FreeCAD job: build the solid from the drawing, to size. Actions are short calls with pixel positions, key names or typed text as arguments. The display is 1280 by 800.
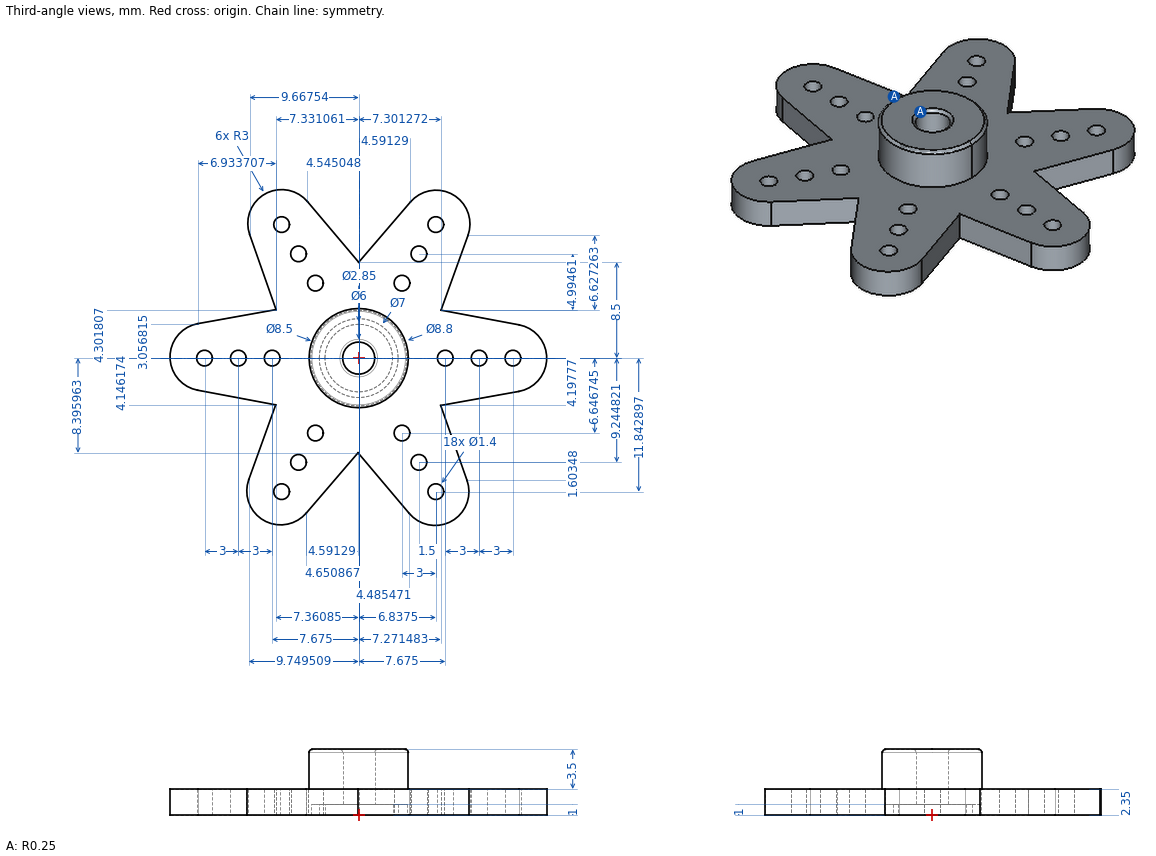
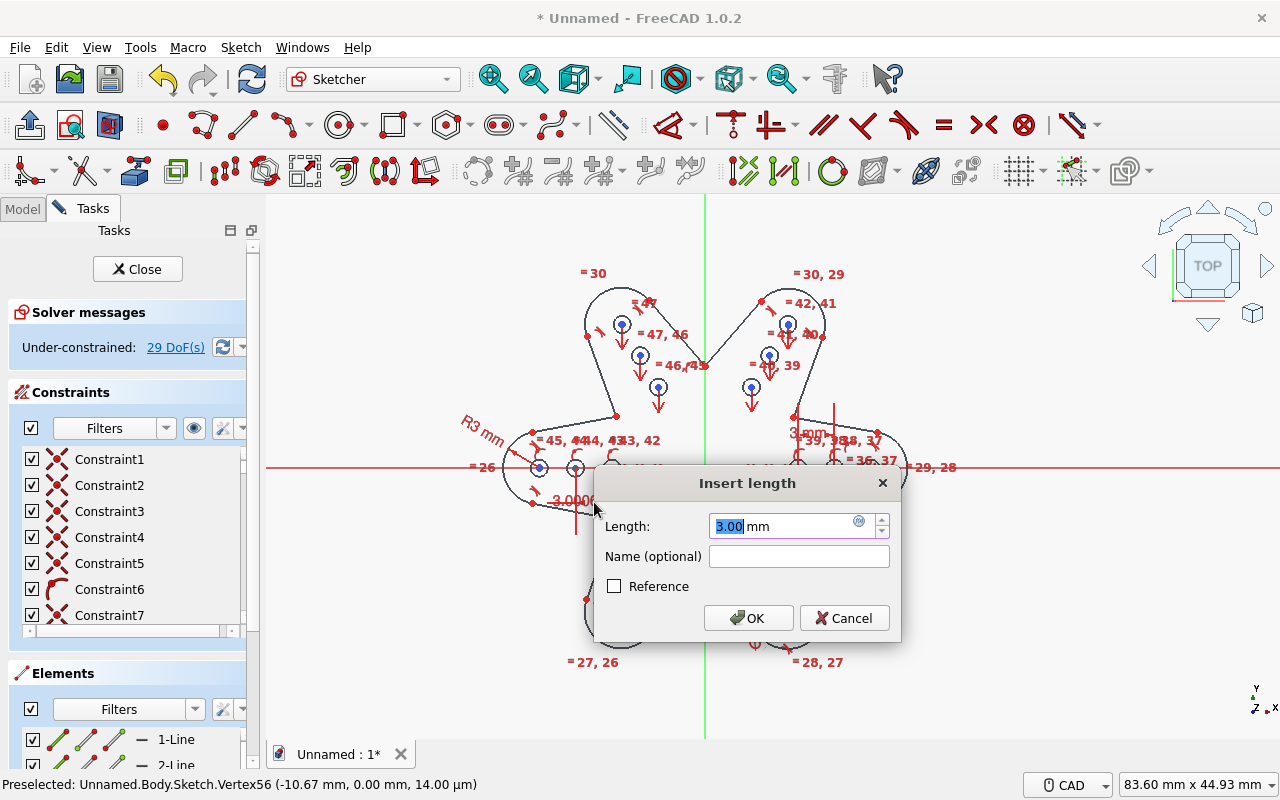
text(3)
key(Return)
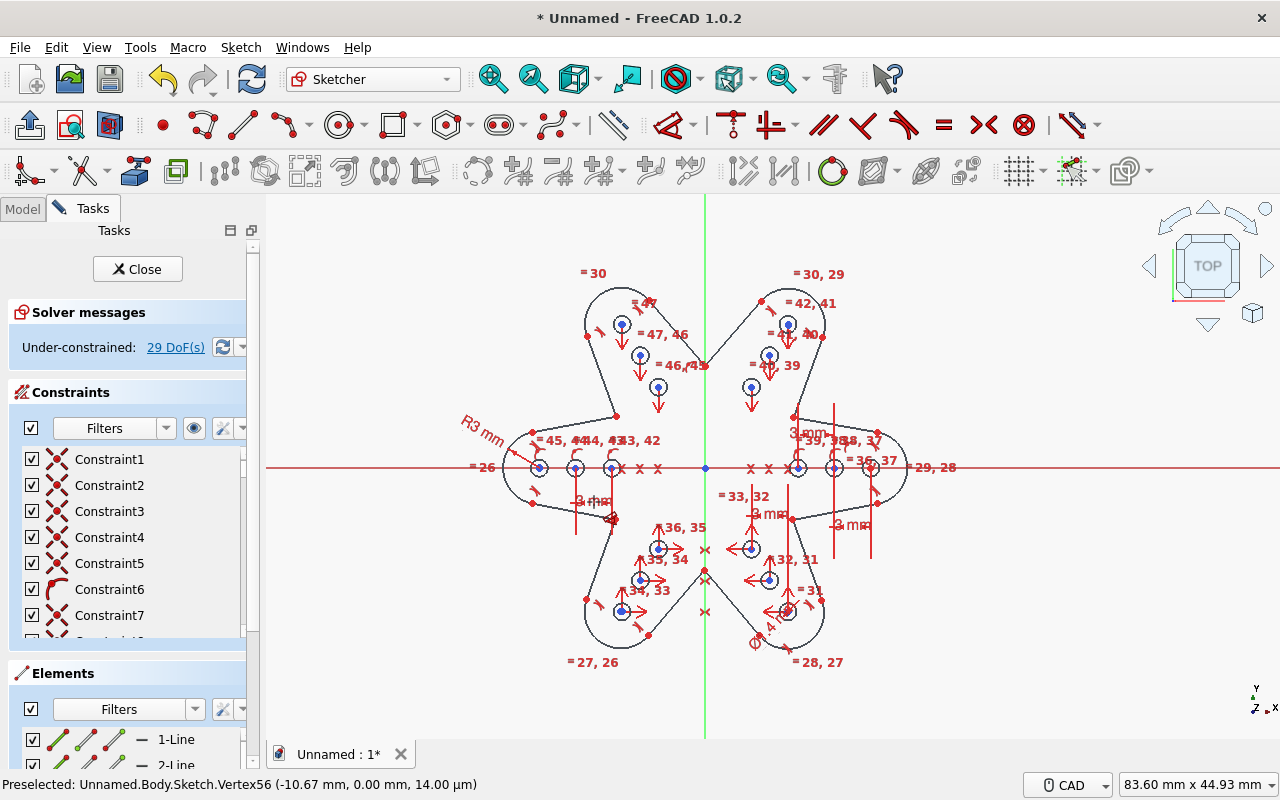
click(576, 468)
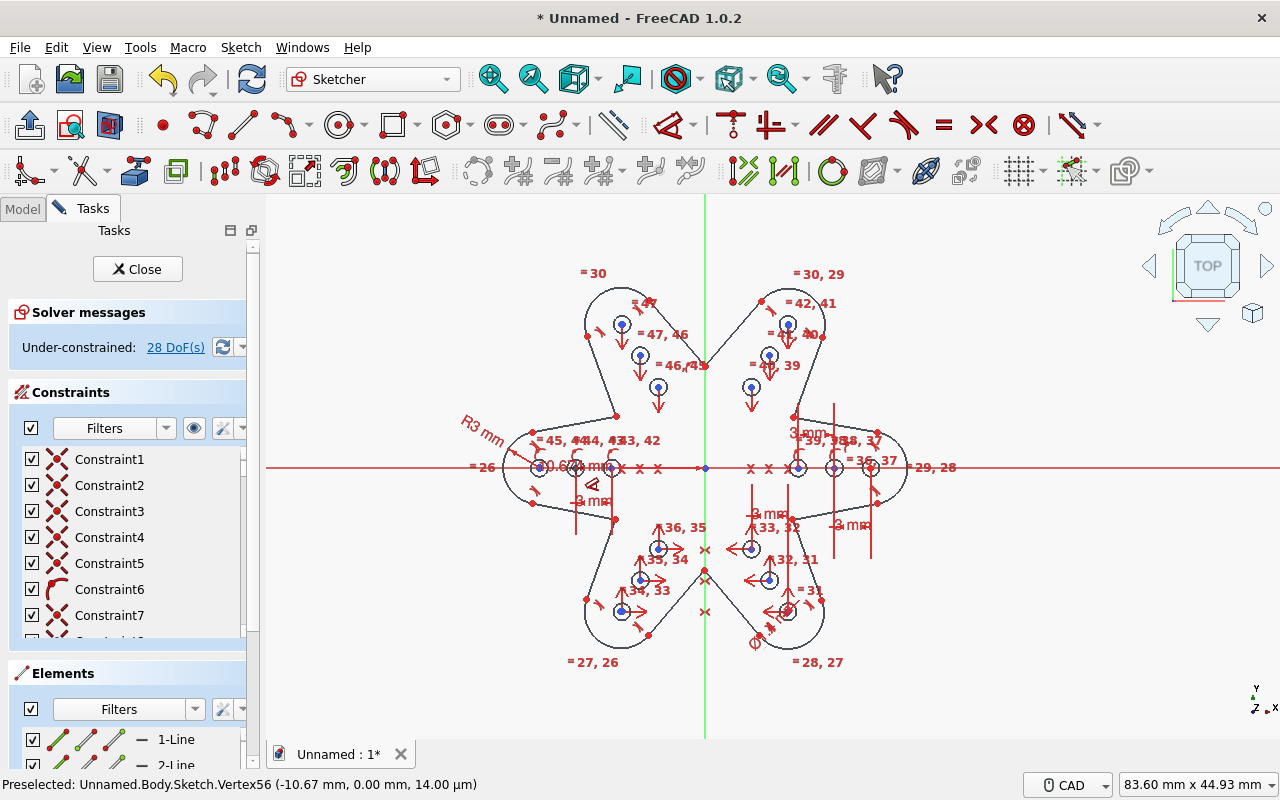
scroll(539, 468, up, 14)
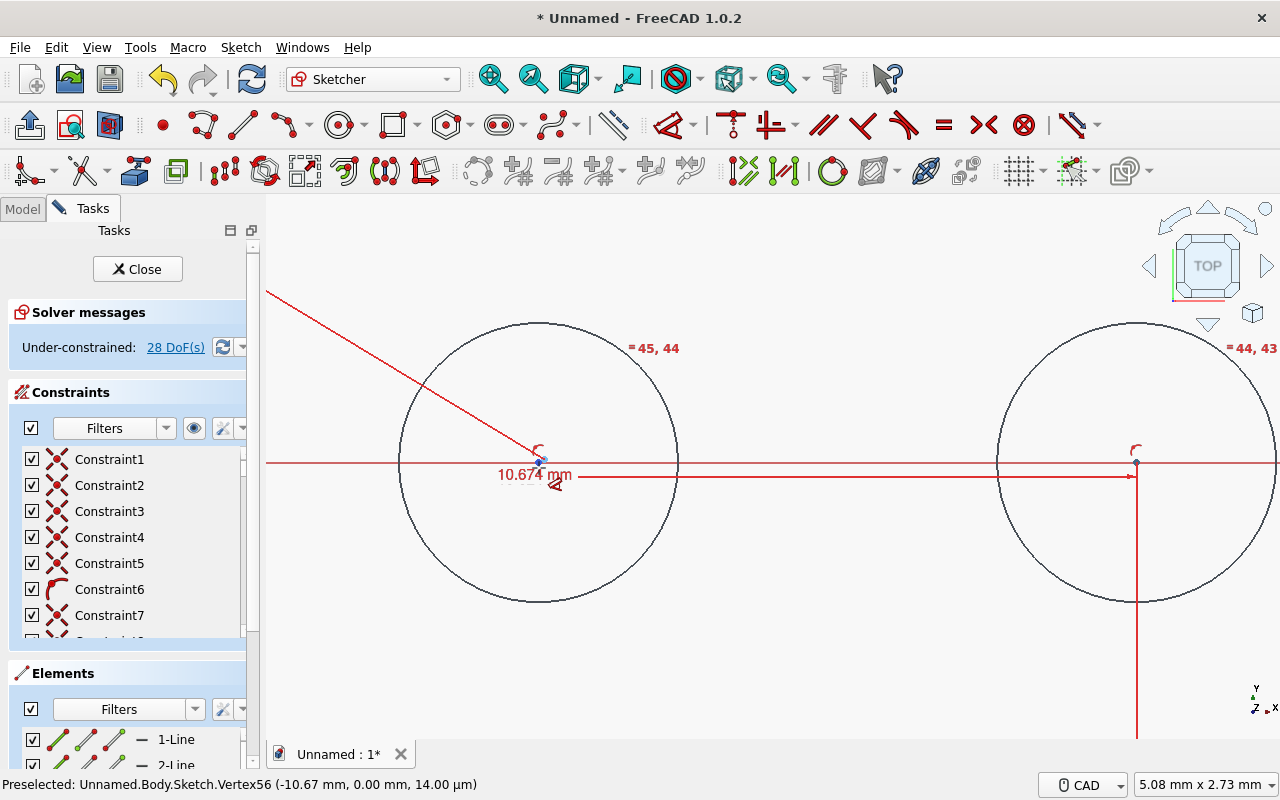
click(538, 463)
click(827, 497)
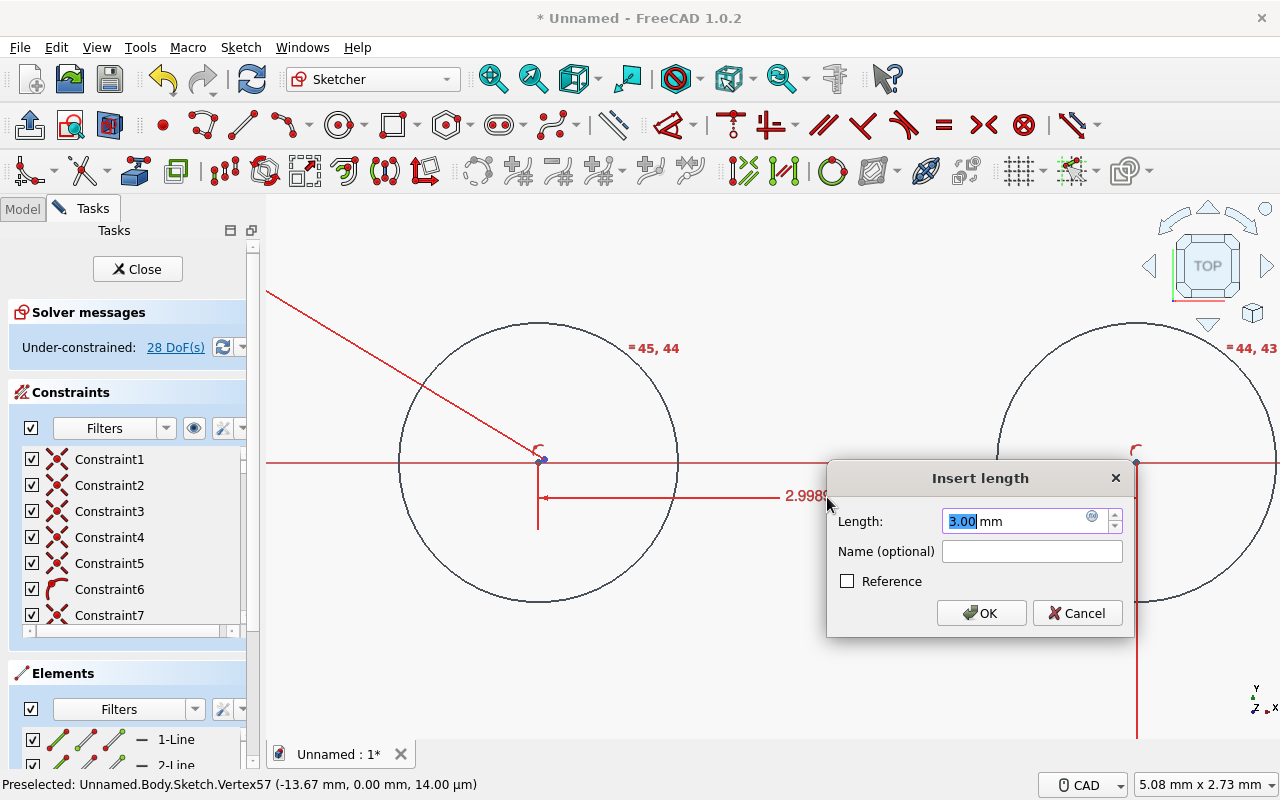
text(3)
key(Return)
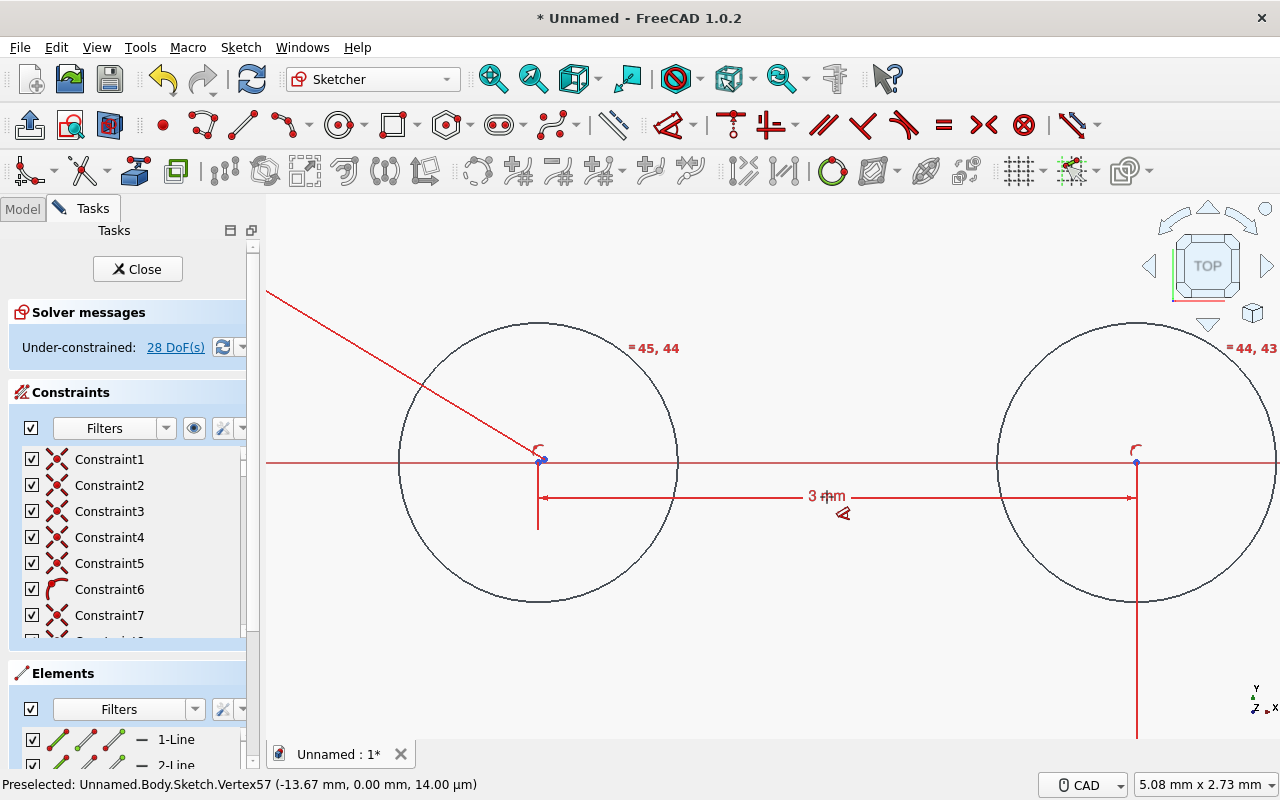
scroll(539, 467, down, 14)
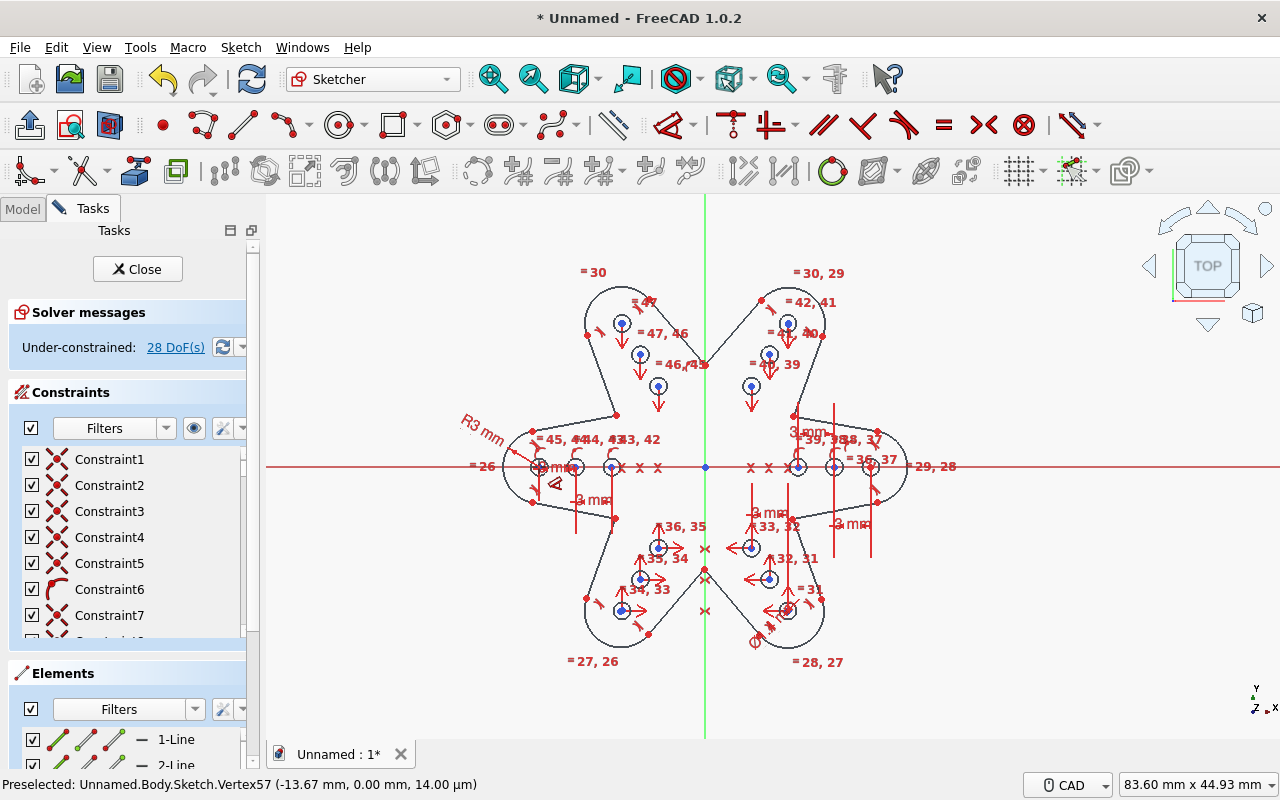
click(705, 365)
click(671, 416)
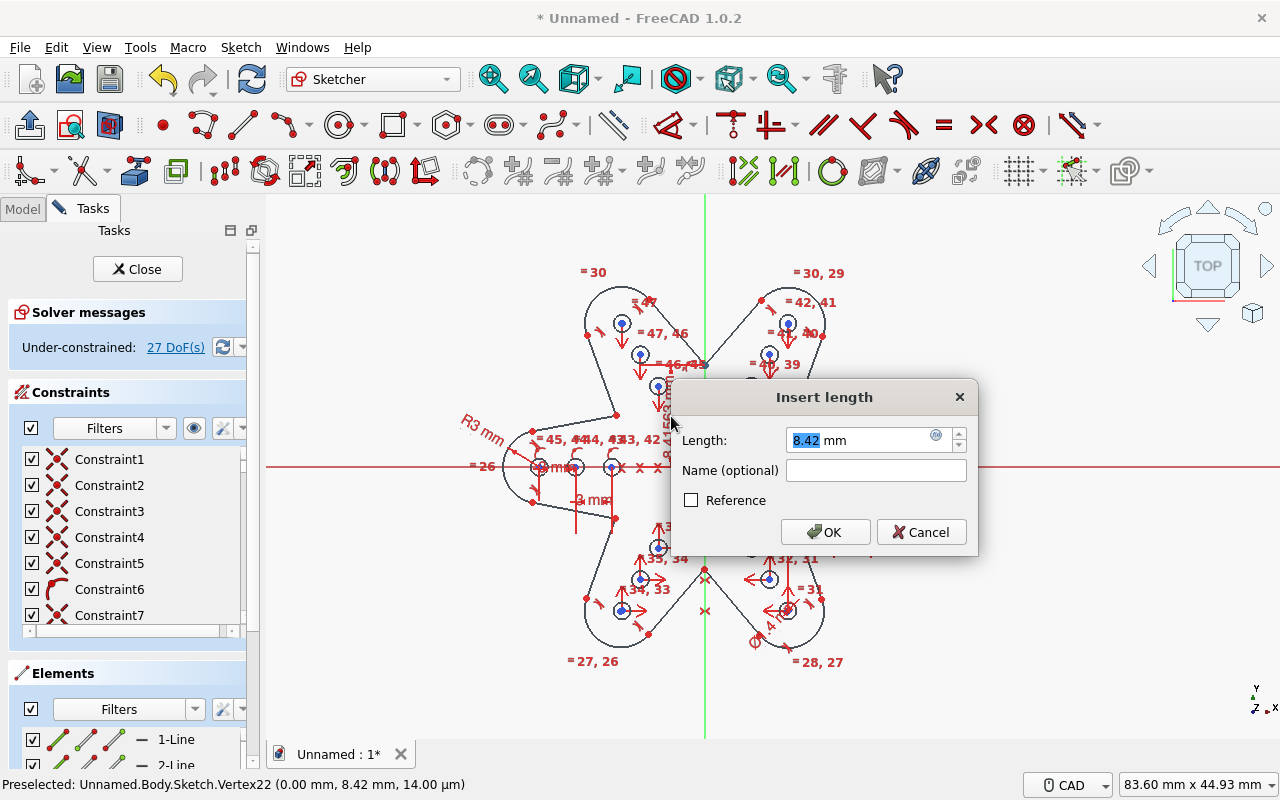
text(8.5)
key(Return)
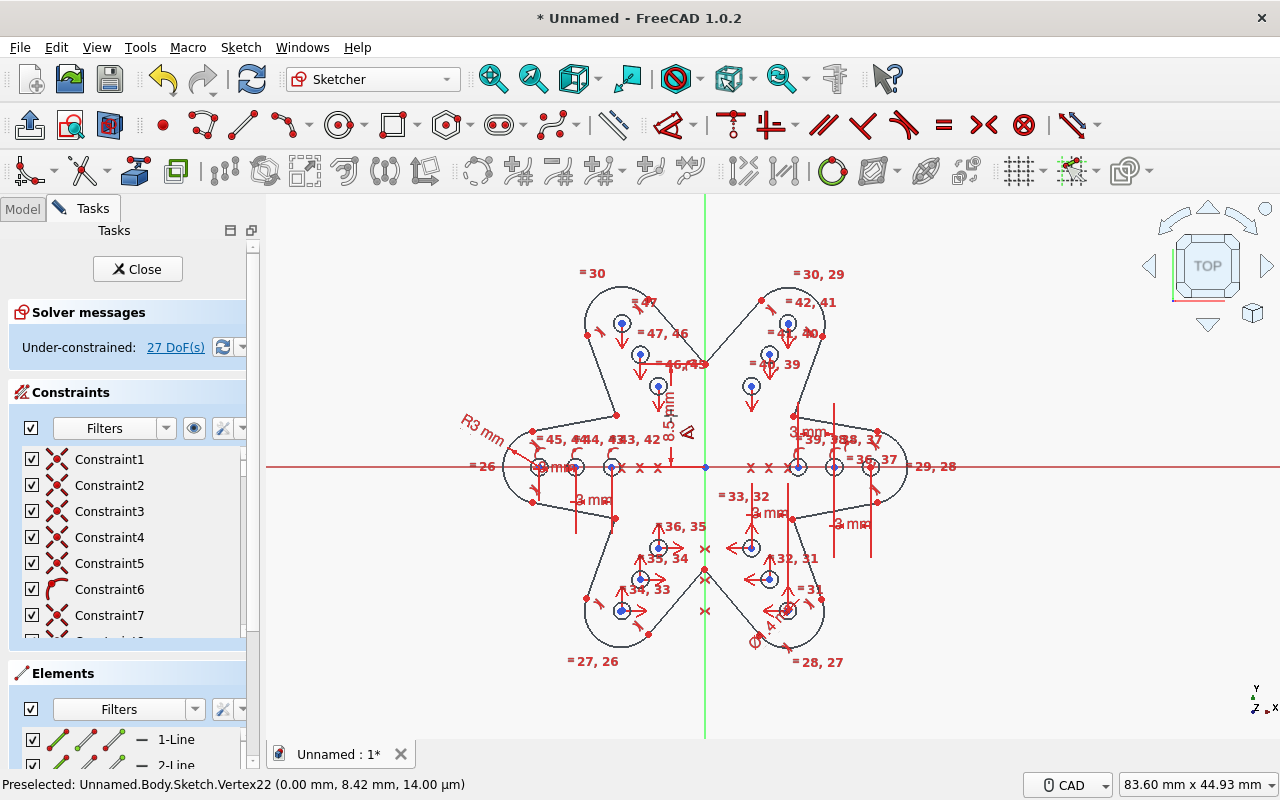
scroll(788, 611, up, 14)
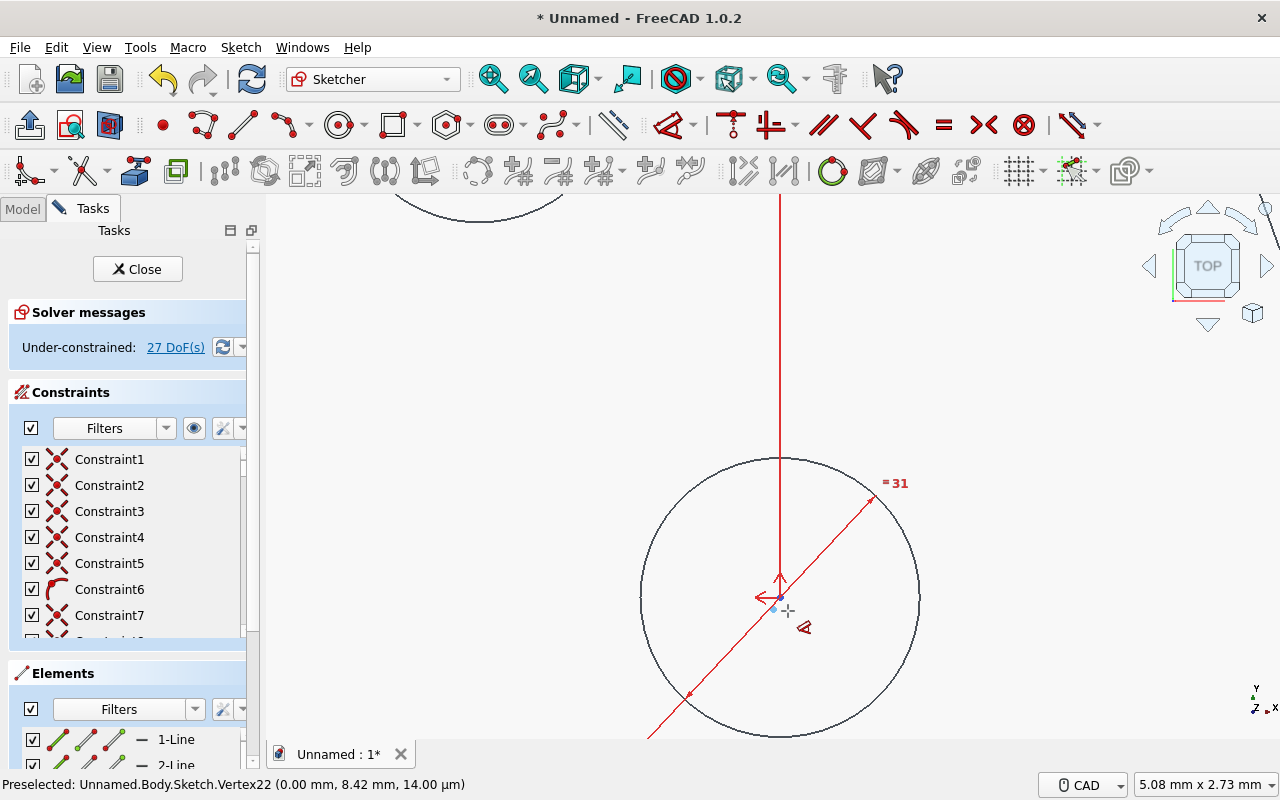
click(780, 598)